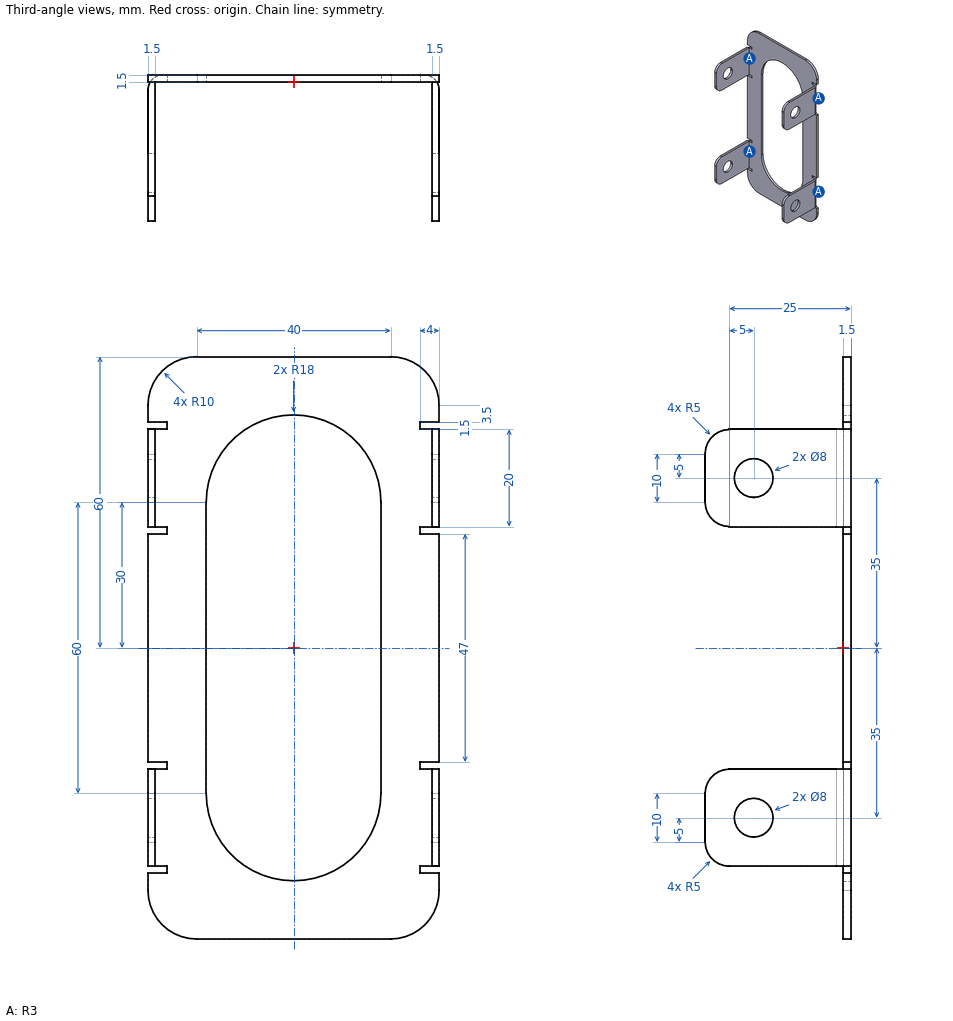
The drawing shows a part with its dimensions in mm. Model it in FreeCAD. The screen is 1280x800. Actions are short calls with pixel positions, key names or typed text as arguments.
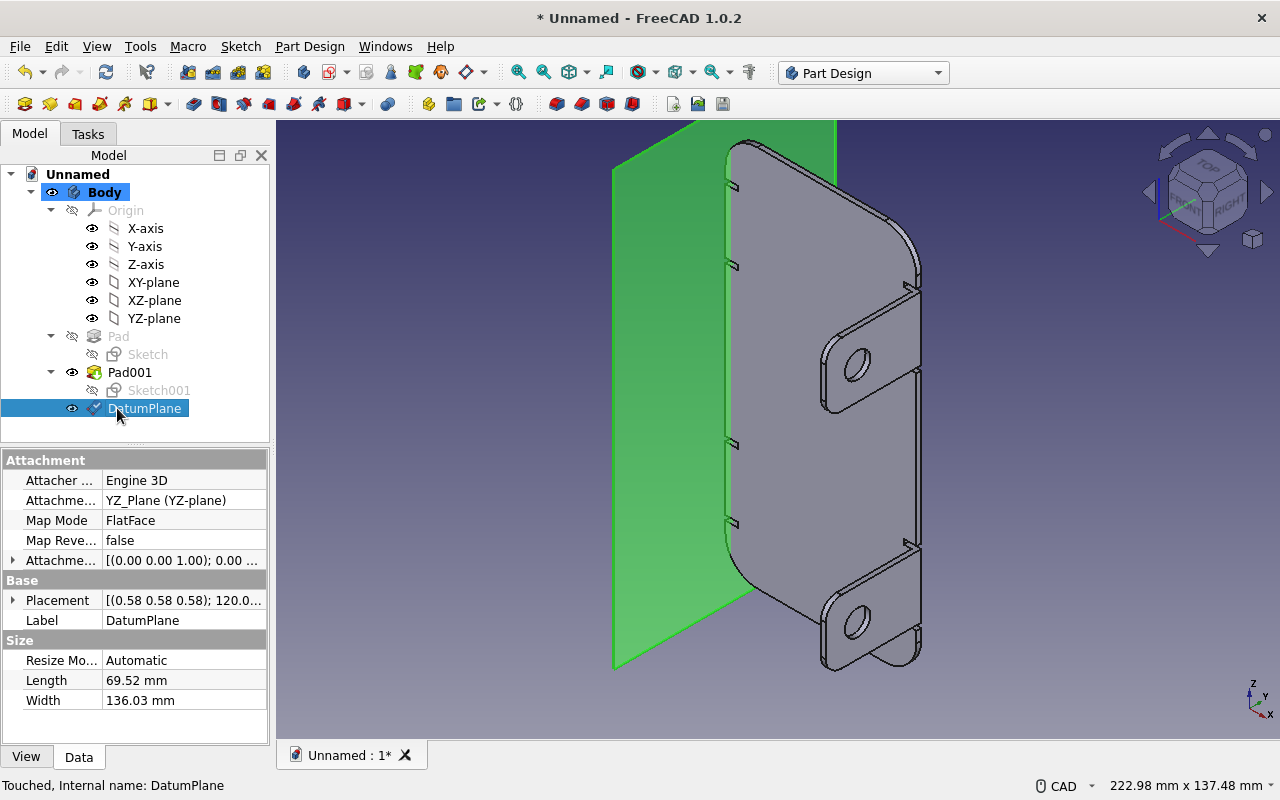
click(328, 72)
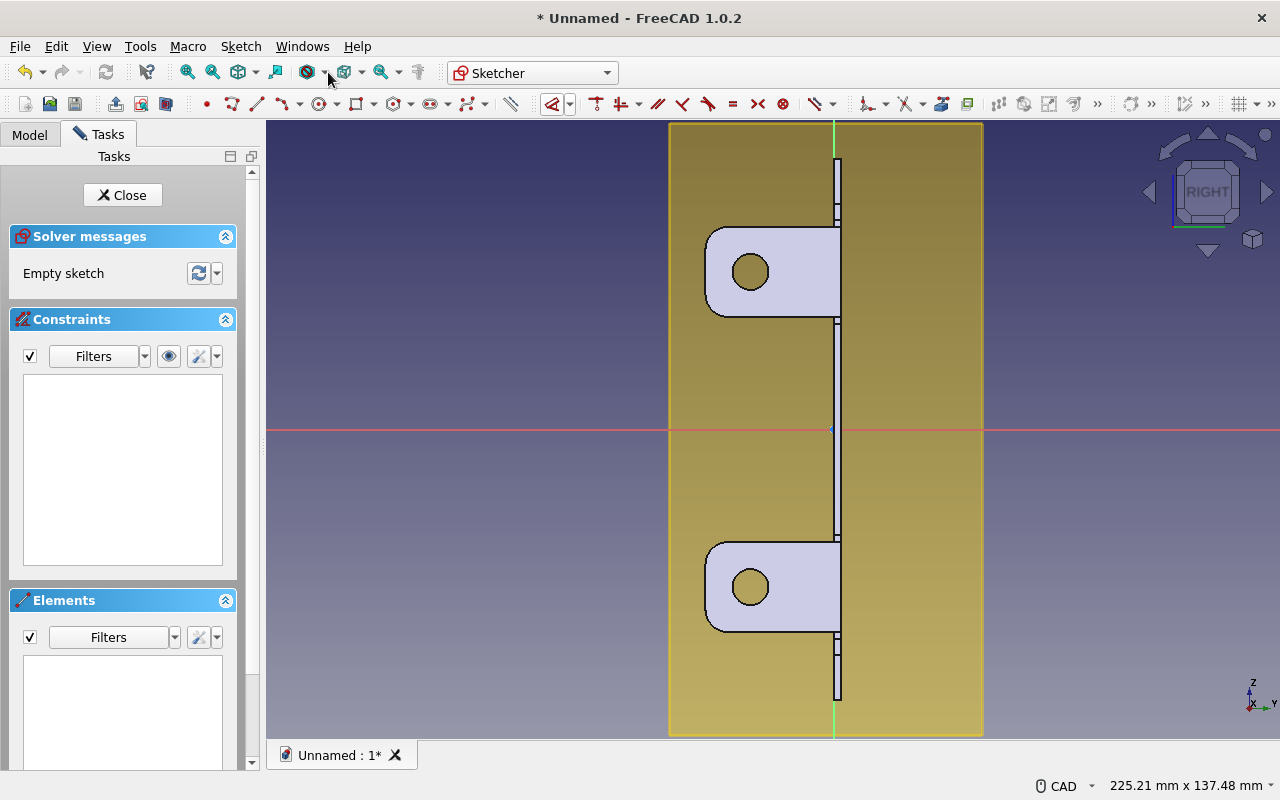
click(166, 104)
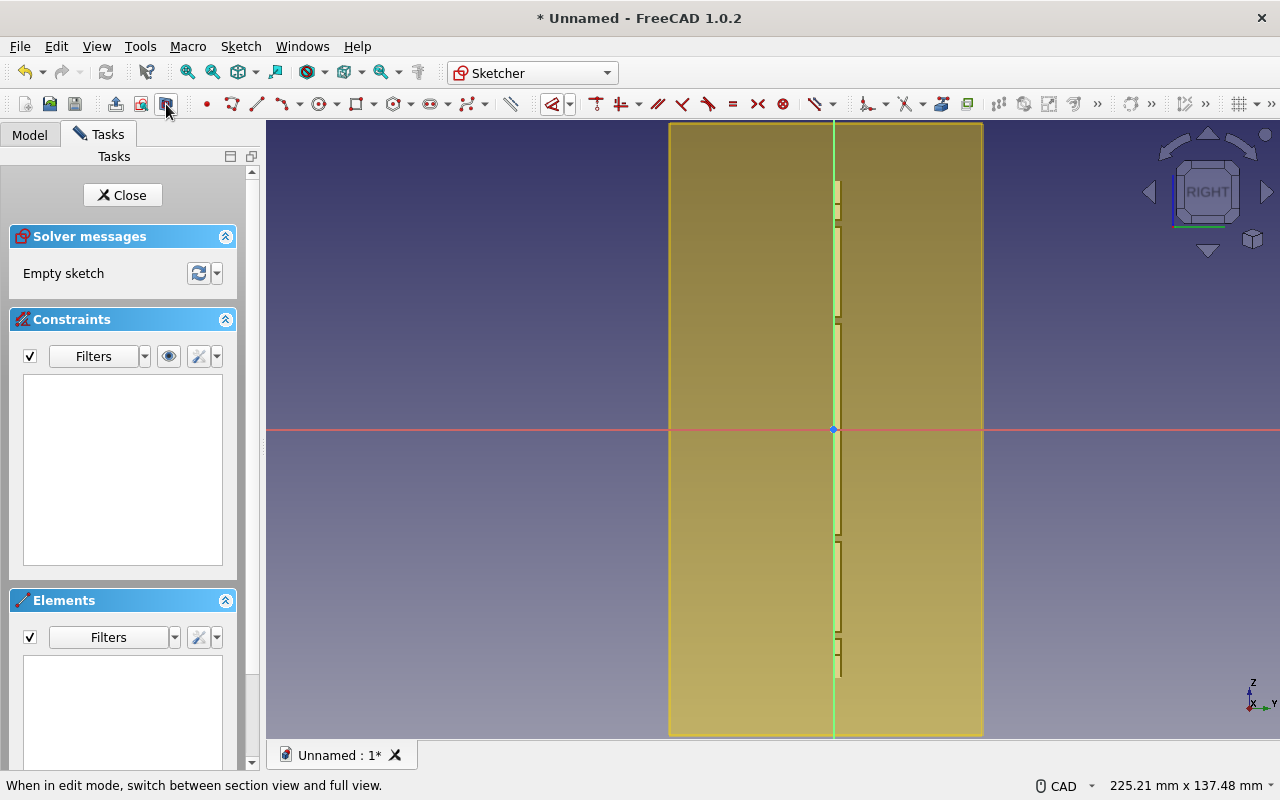
click(257, 104)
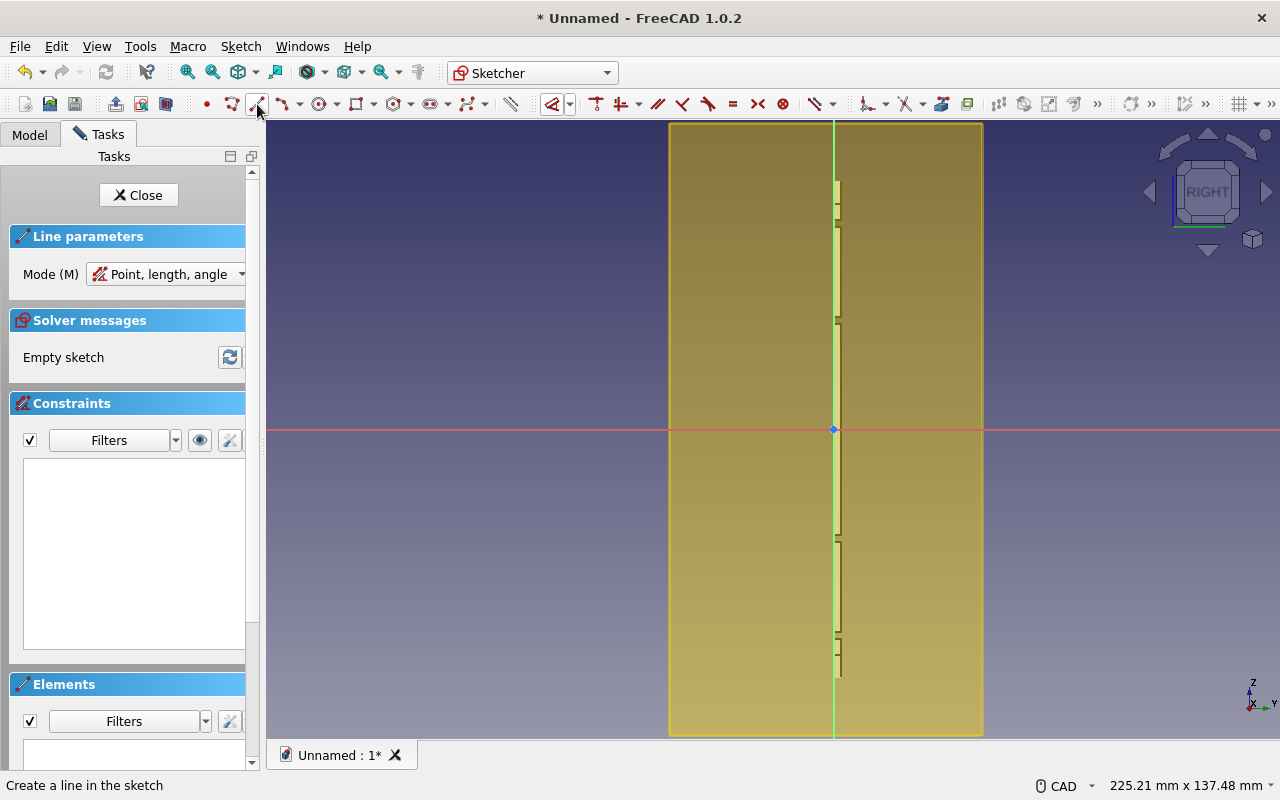
click(705, 610)
click(705, 565)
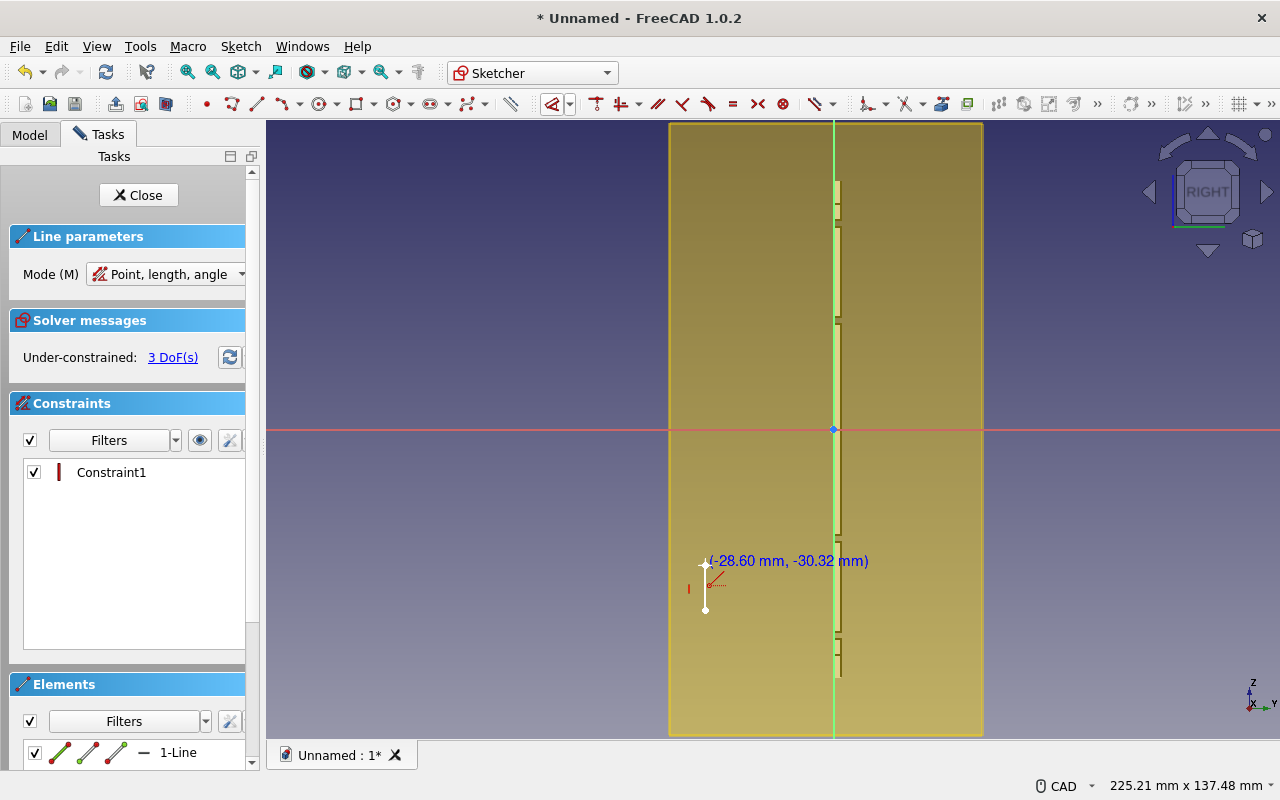
click(232, 104)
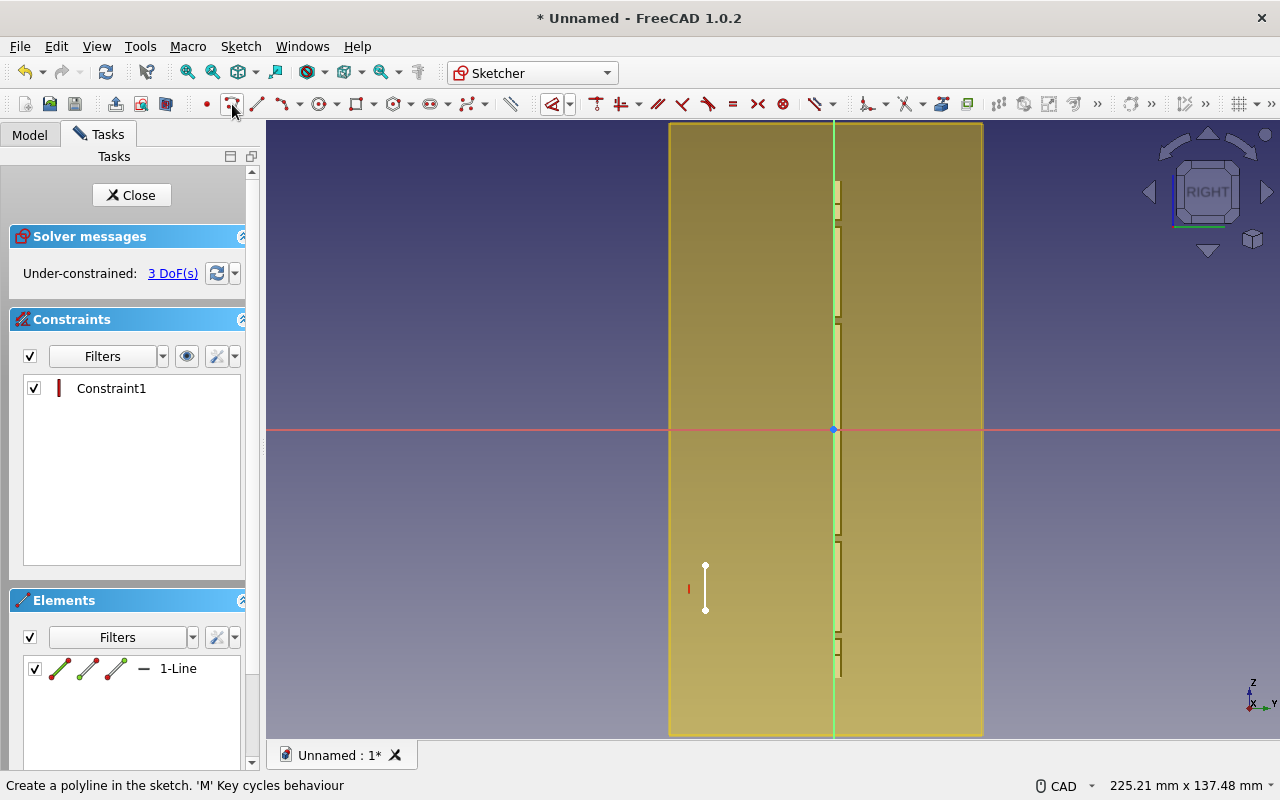
click(728, 542)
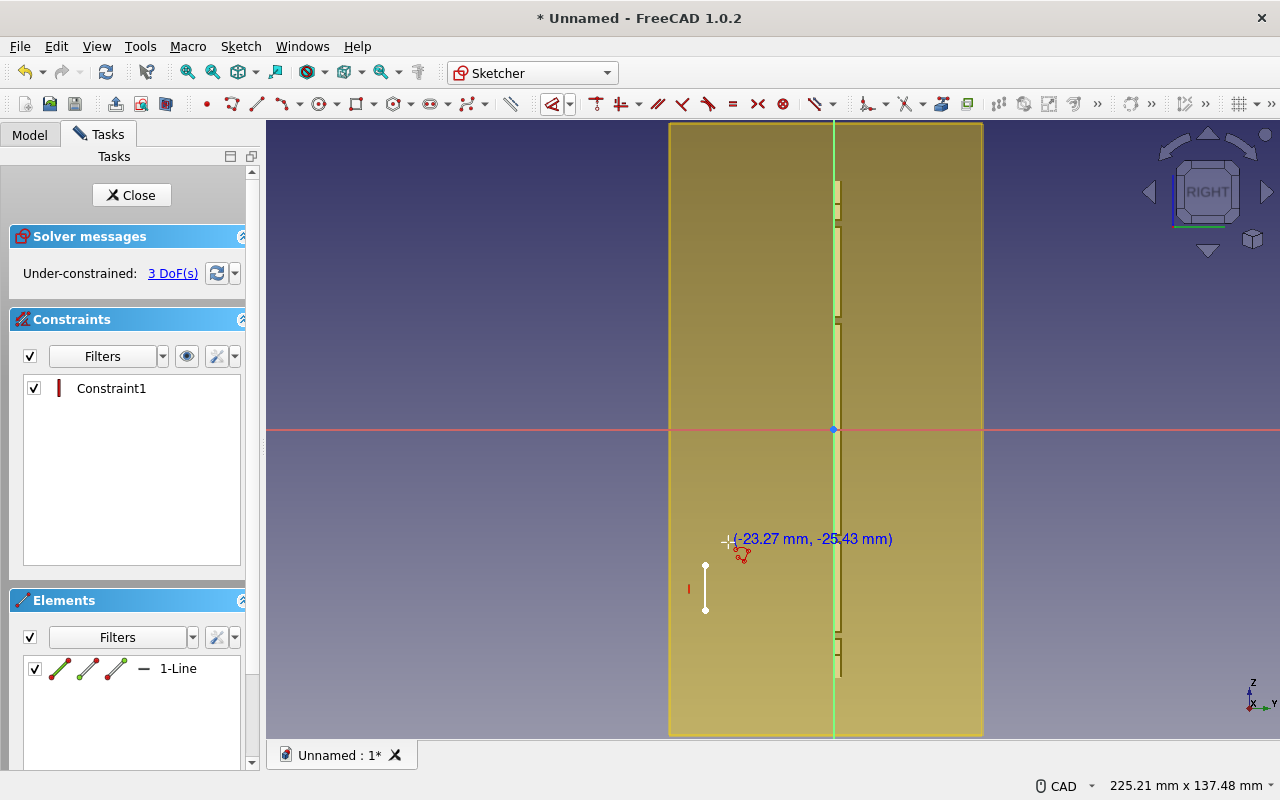
scroll(841, 542, up, 5)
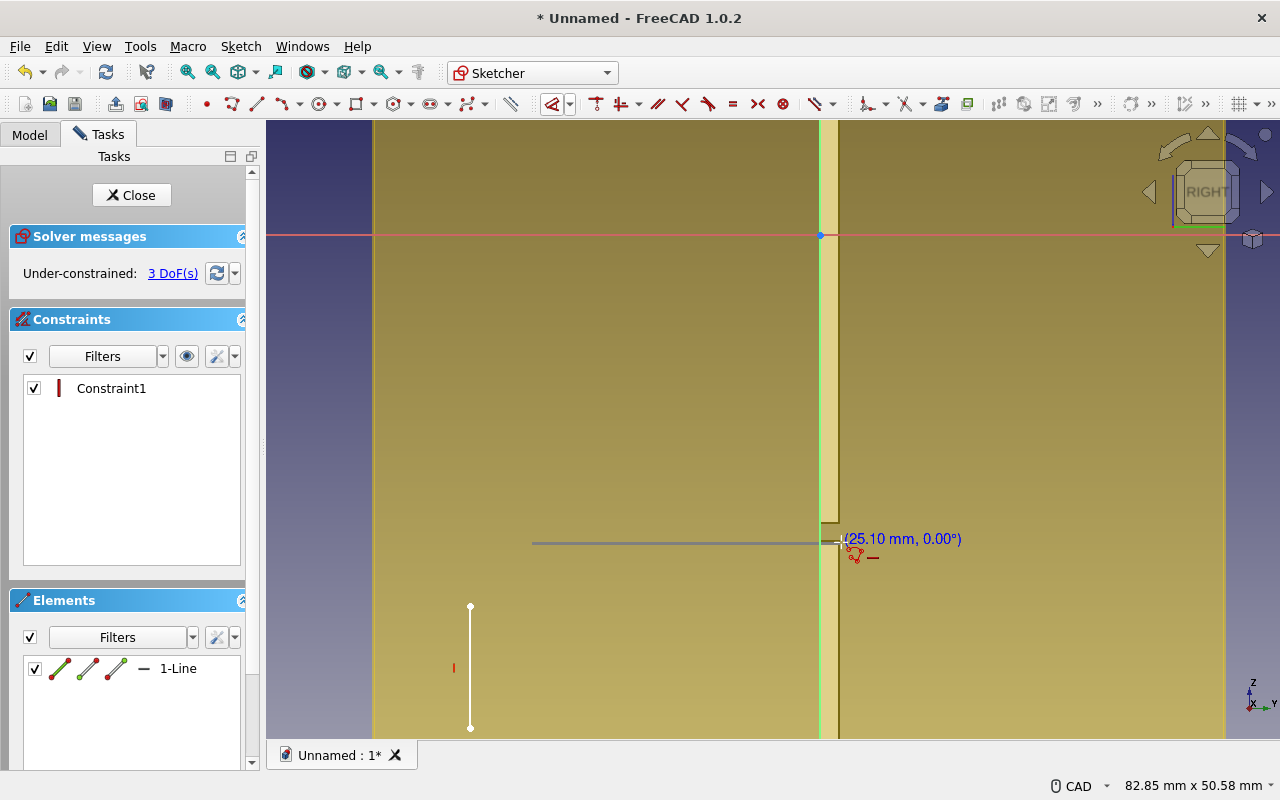
click(839, 541)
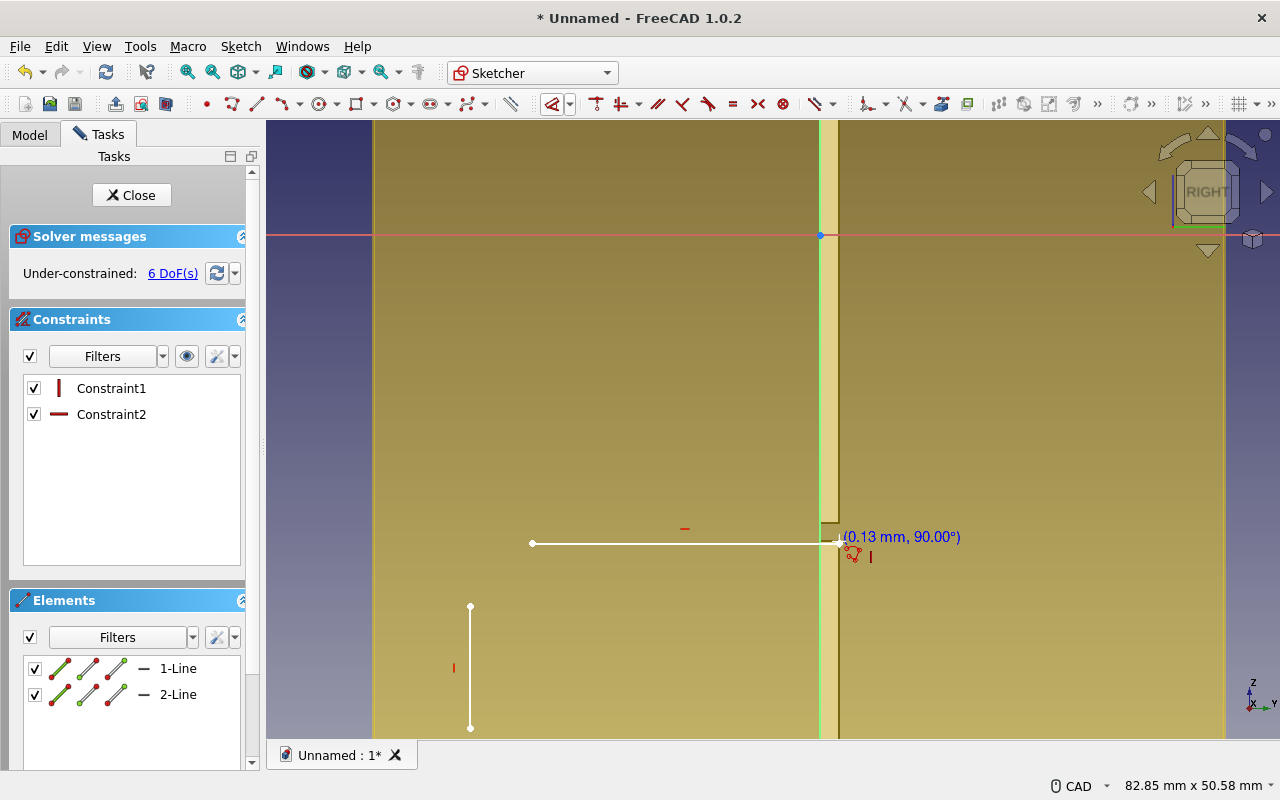
scroll(733, 543, down, 5)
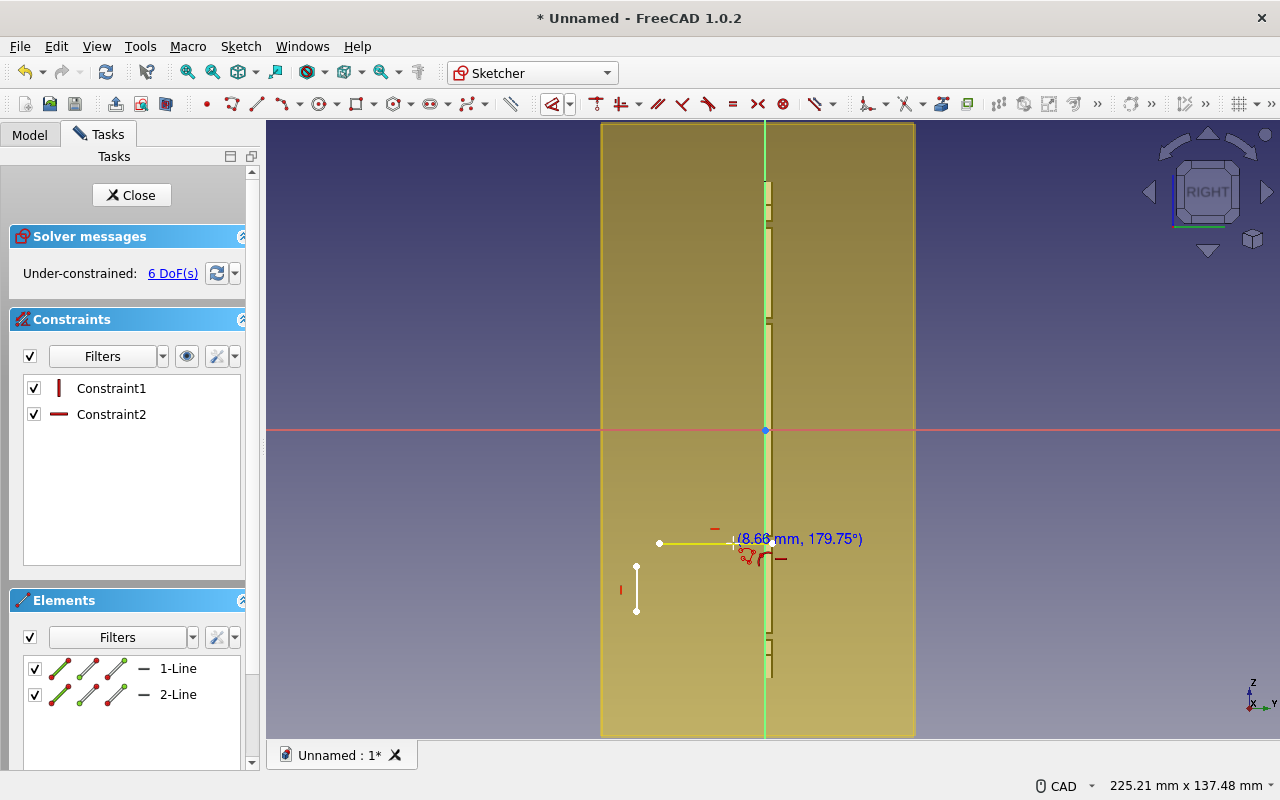
scroll(772, 633, up, 5)